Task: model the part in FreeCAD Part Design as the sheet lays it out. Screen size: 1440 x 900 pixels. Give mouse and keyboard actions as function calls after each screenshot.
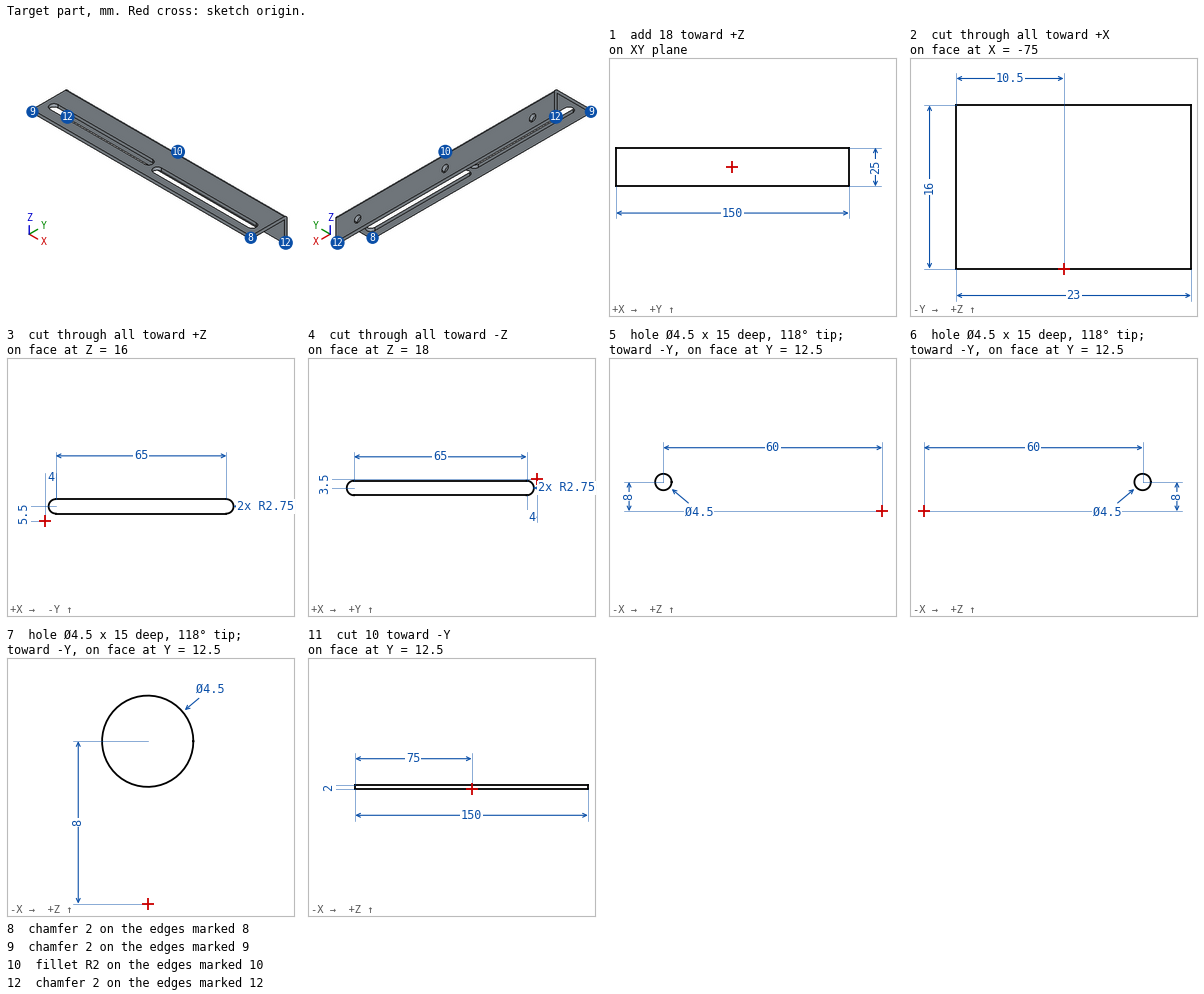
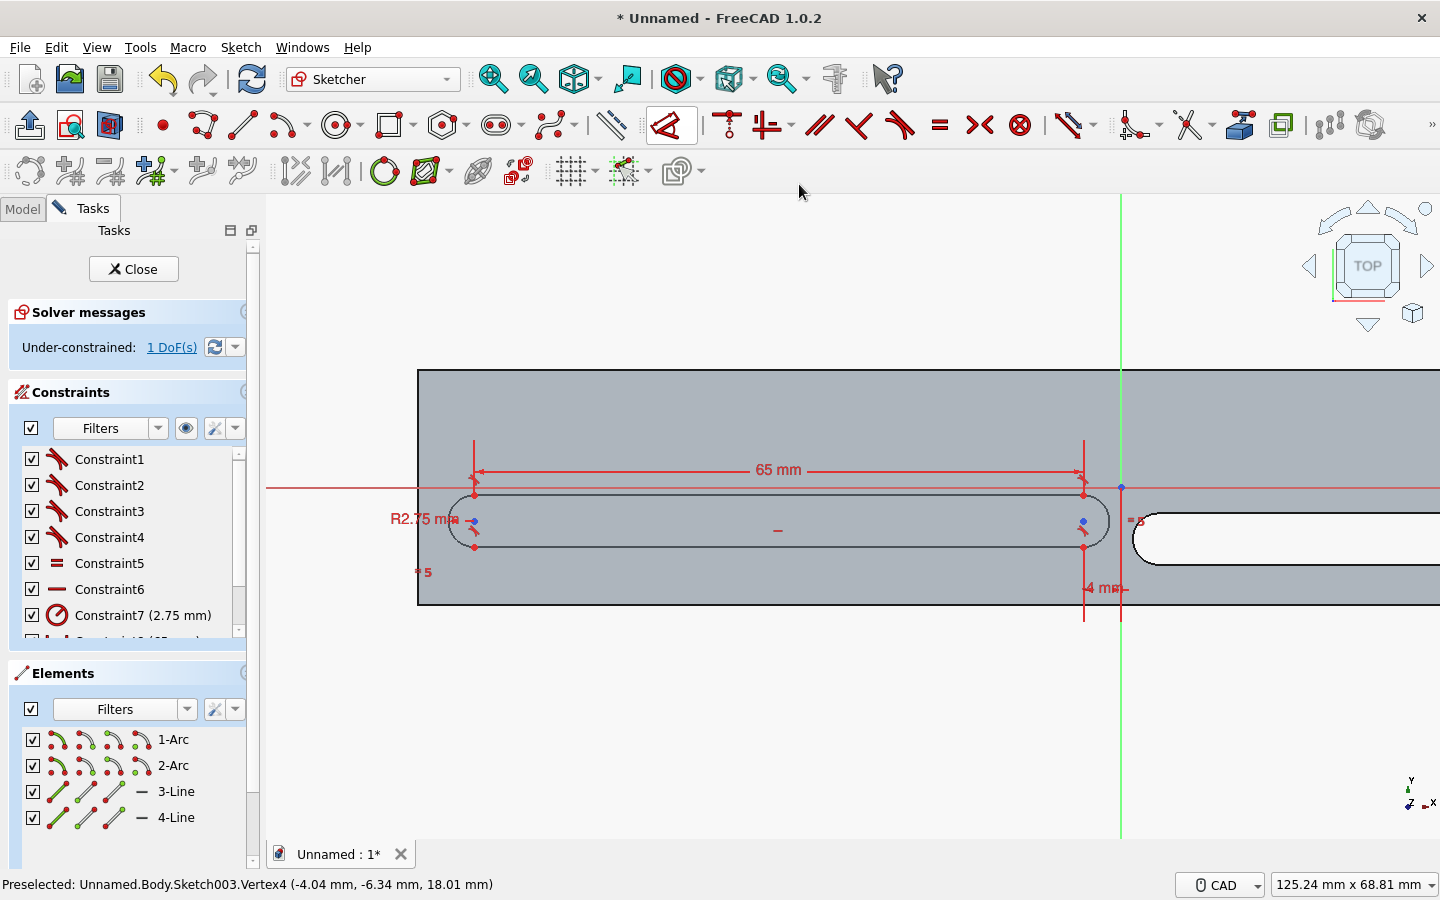
click(474, 521)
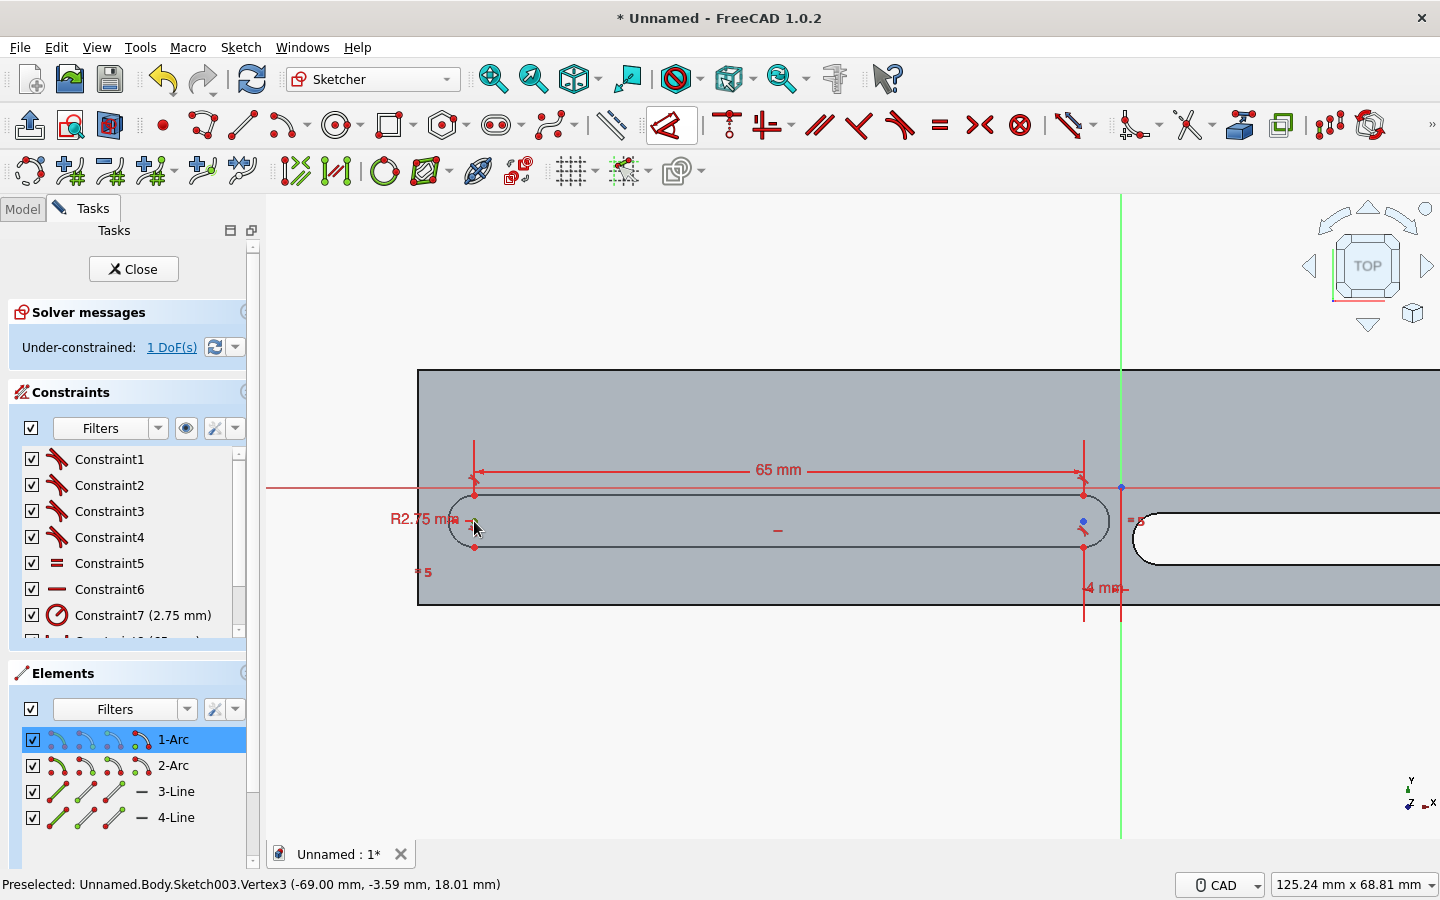
click(692, 126)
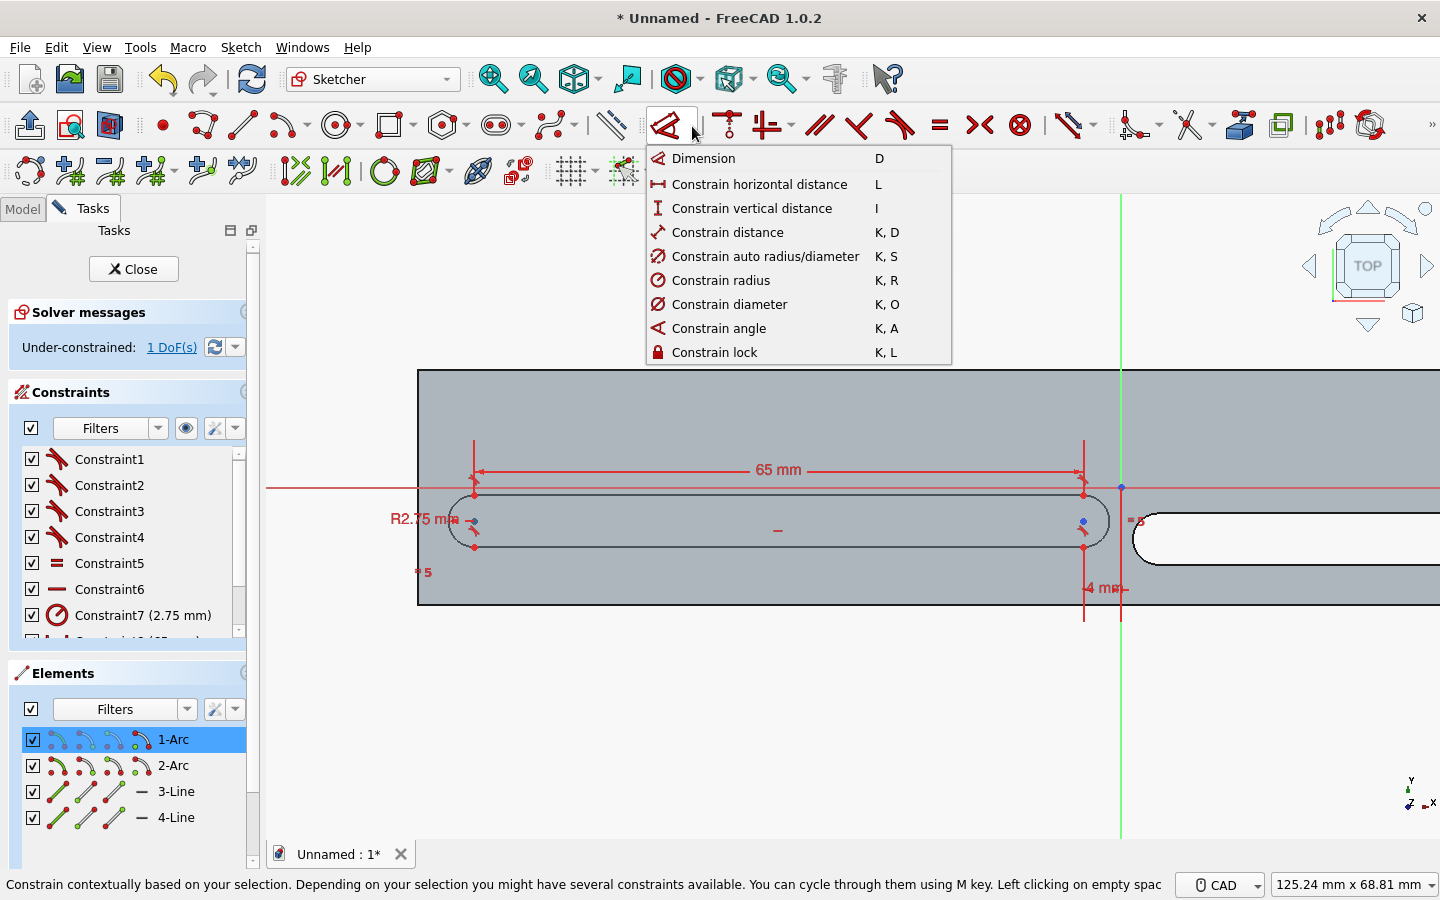
click(799, 208)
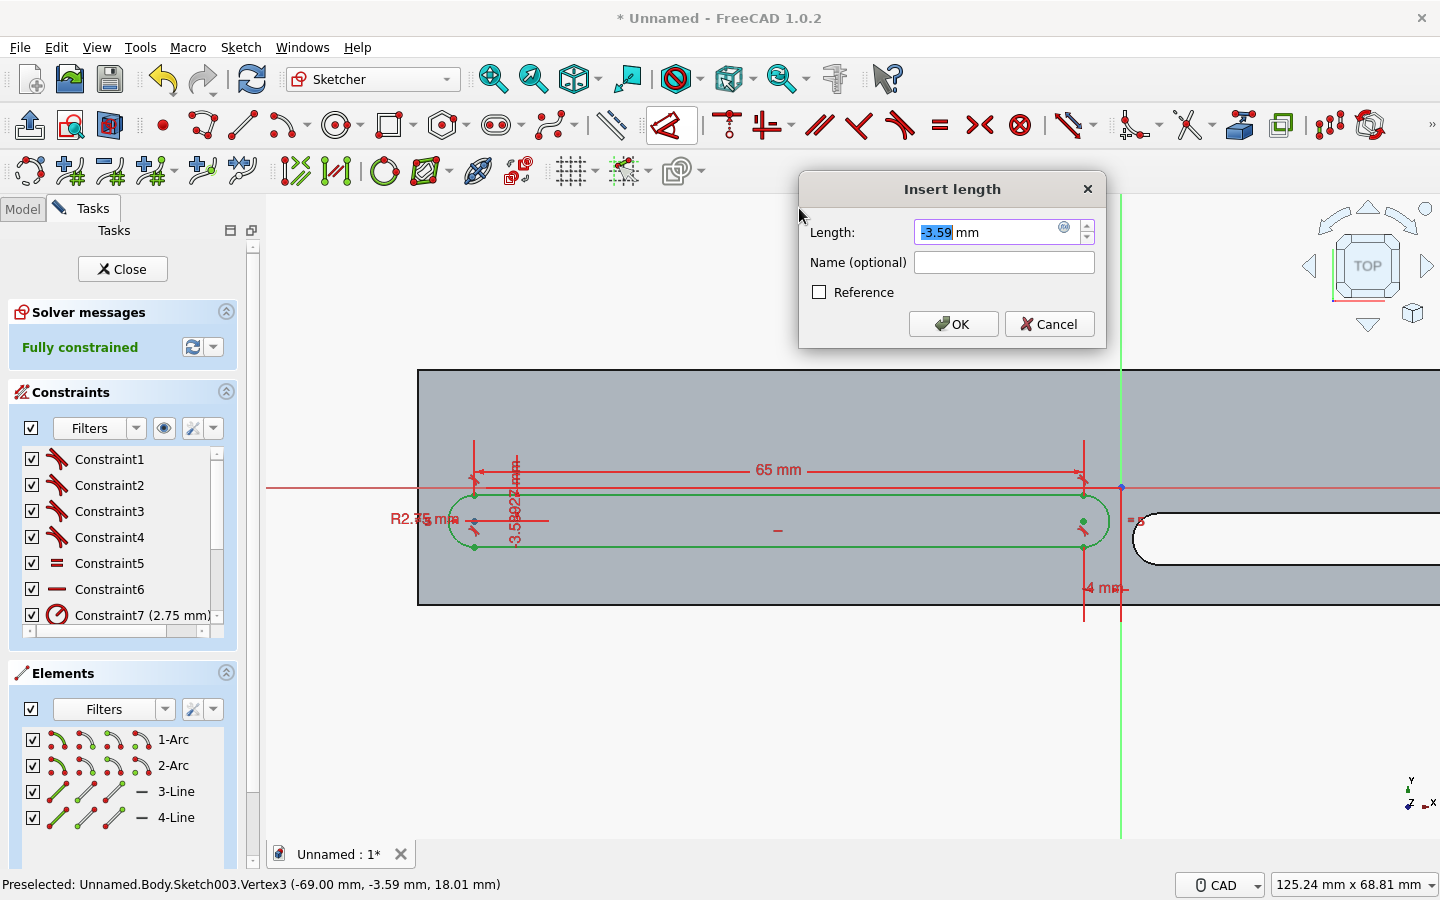
text(-3.5)
key(Return)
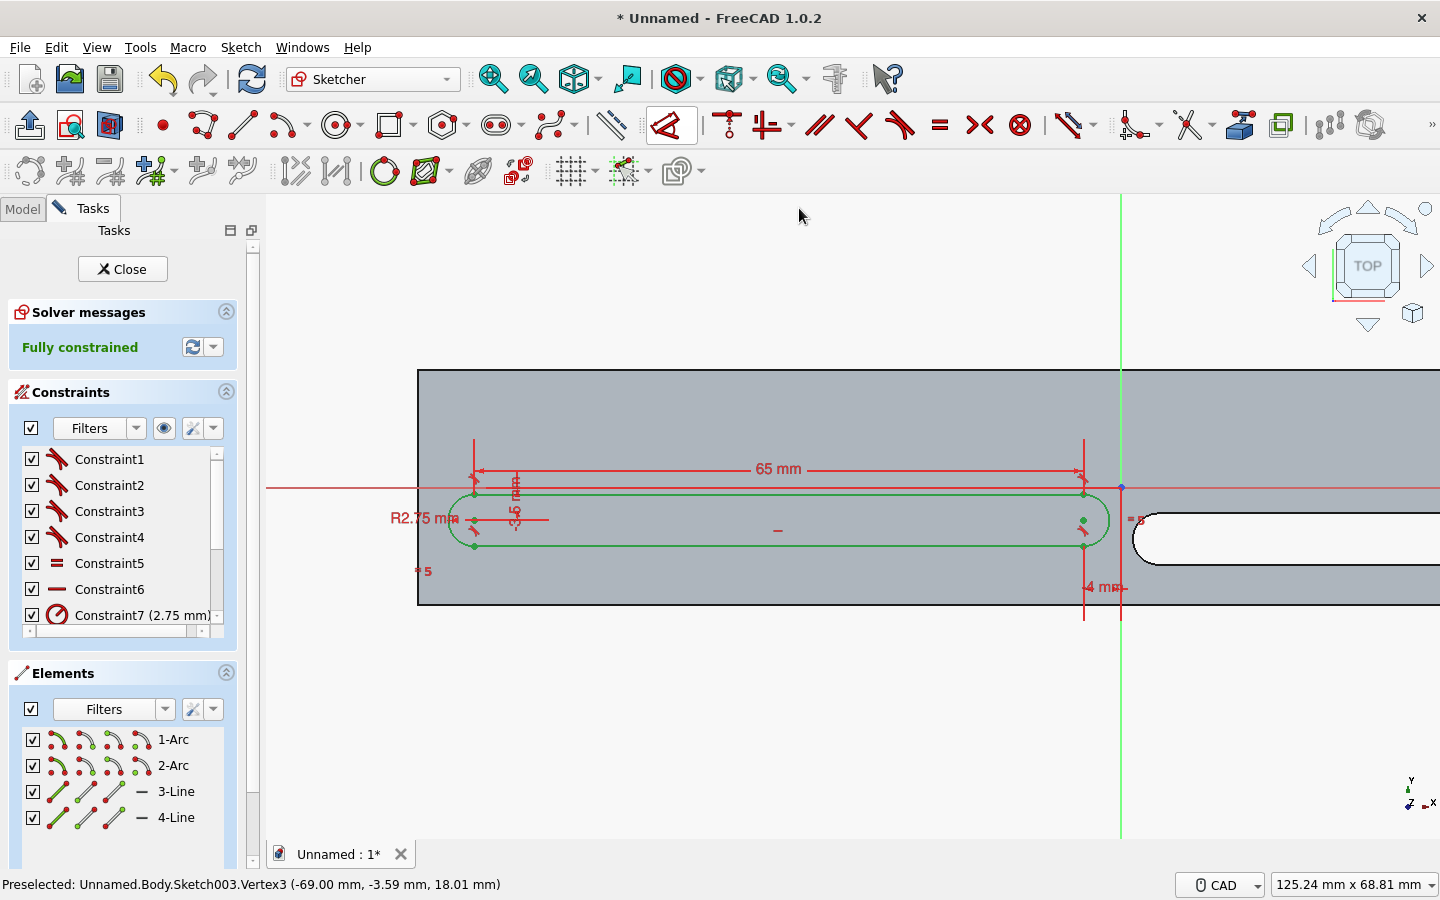
click(123, 269)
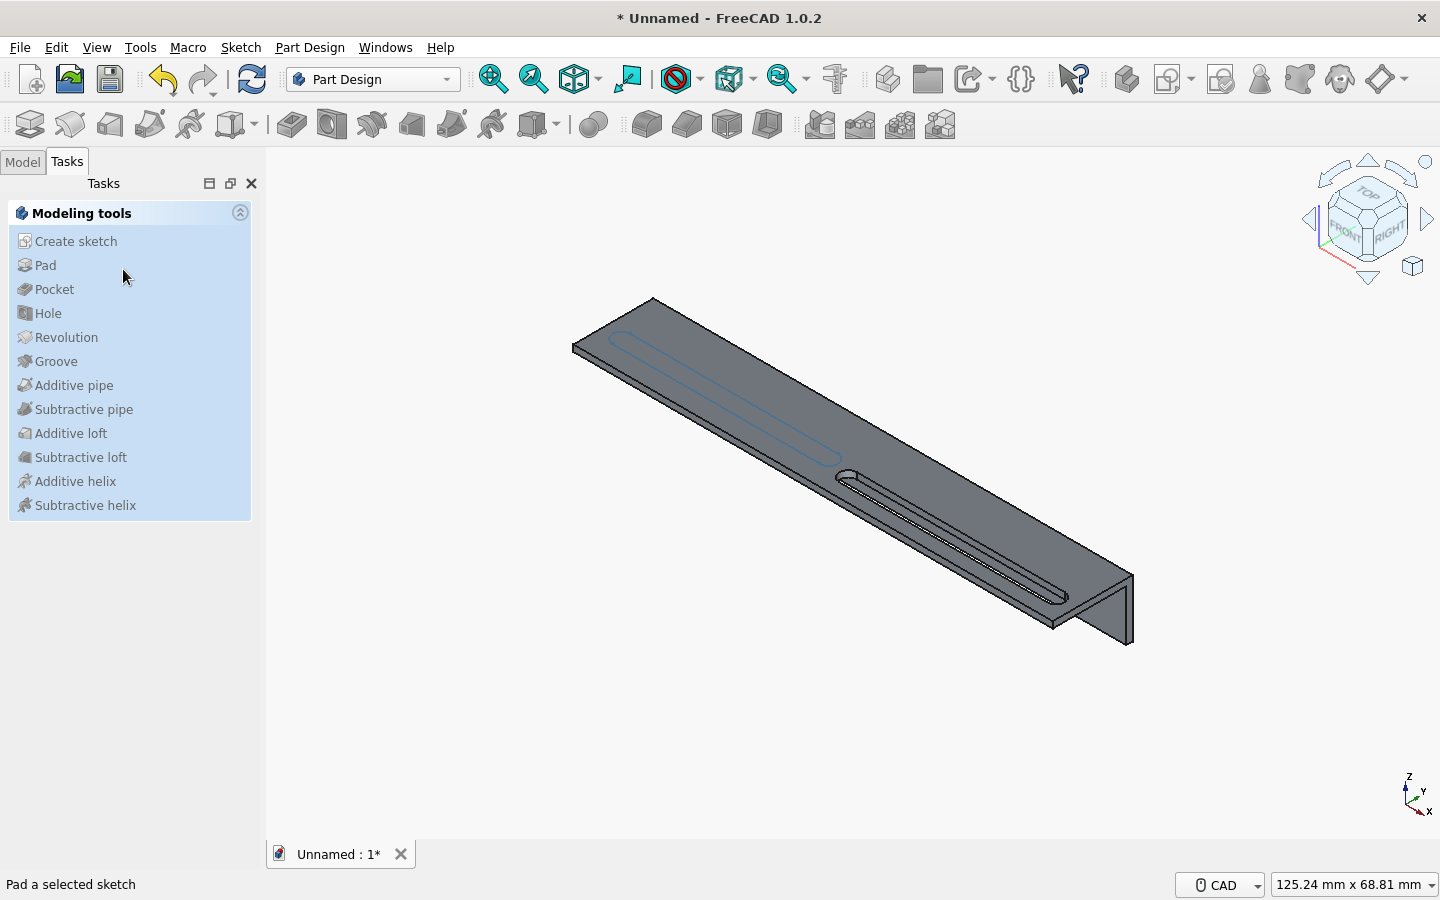
click(292, 124)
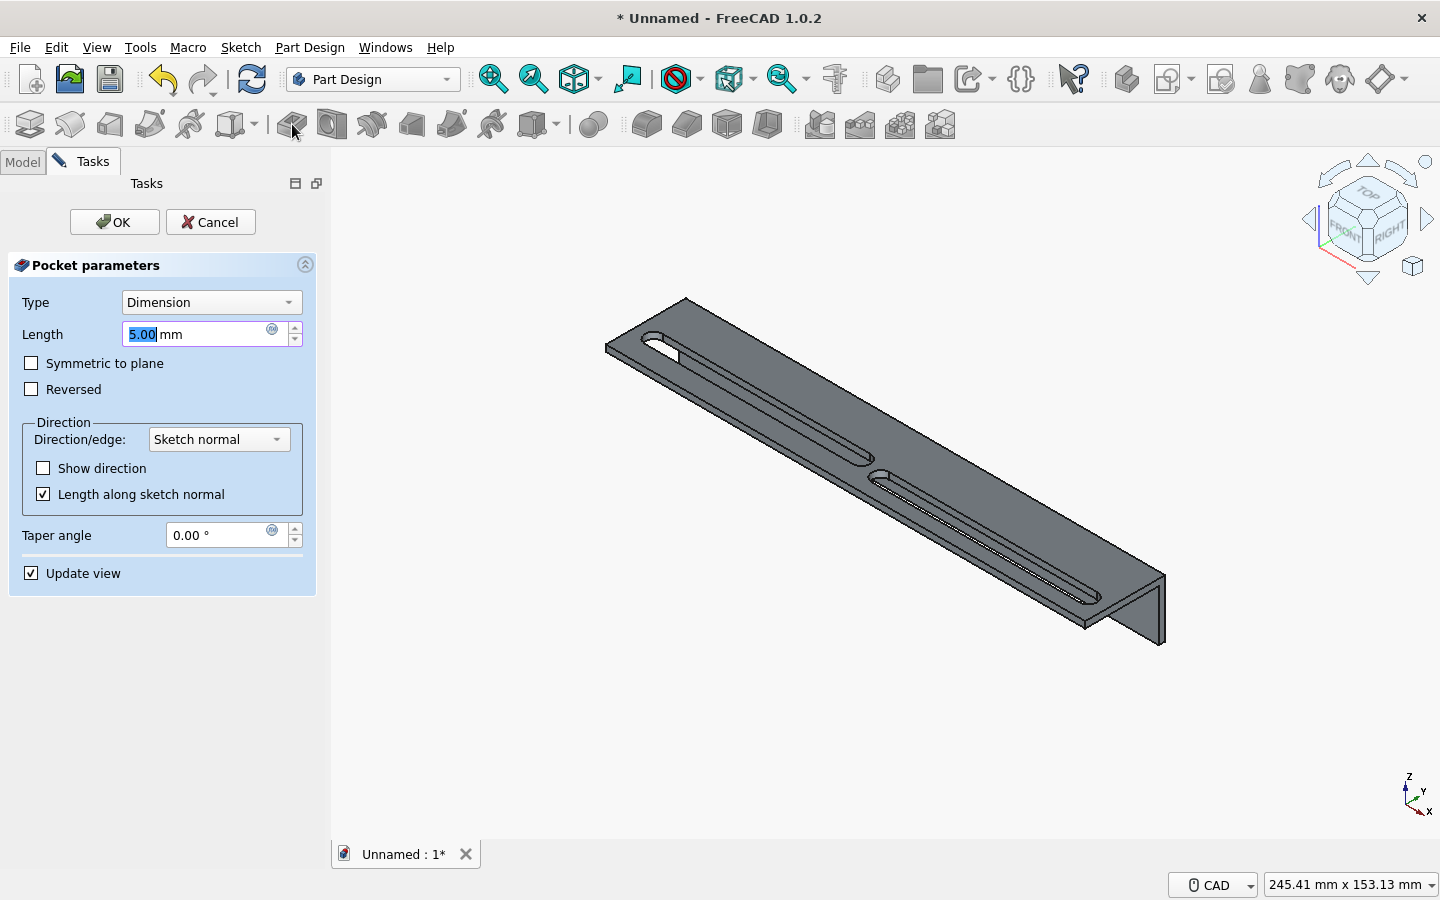
click(212, 302)